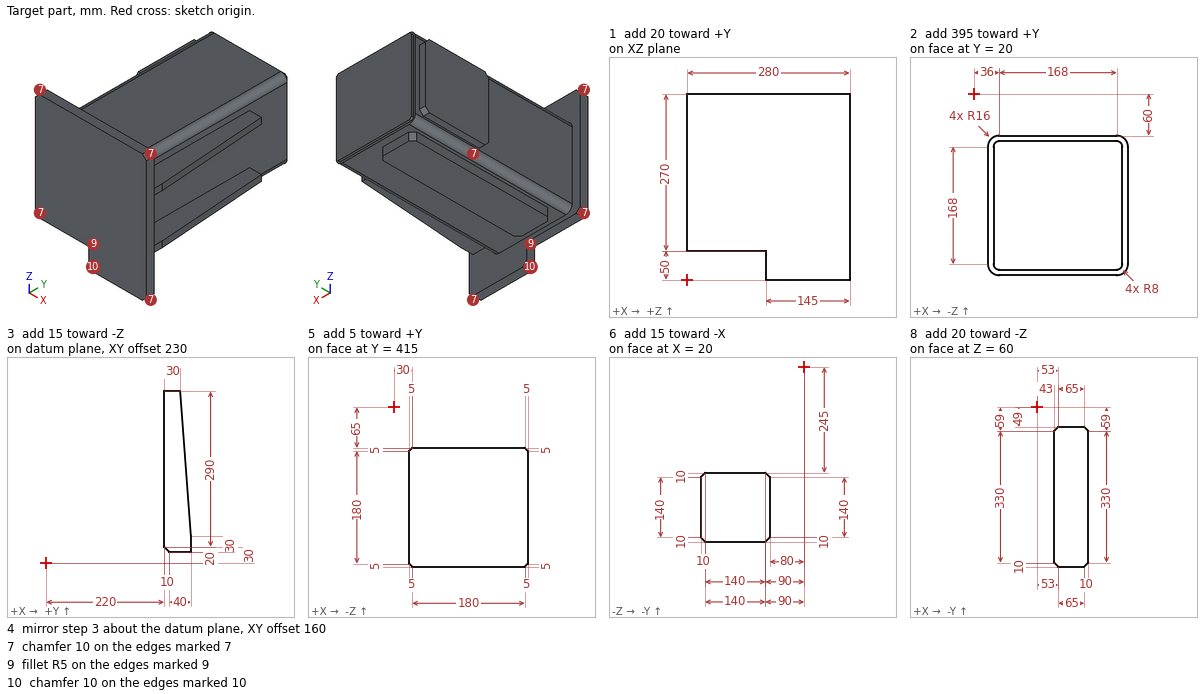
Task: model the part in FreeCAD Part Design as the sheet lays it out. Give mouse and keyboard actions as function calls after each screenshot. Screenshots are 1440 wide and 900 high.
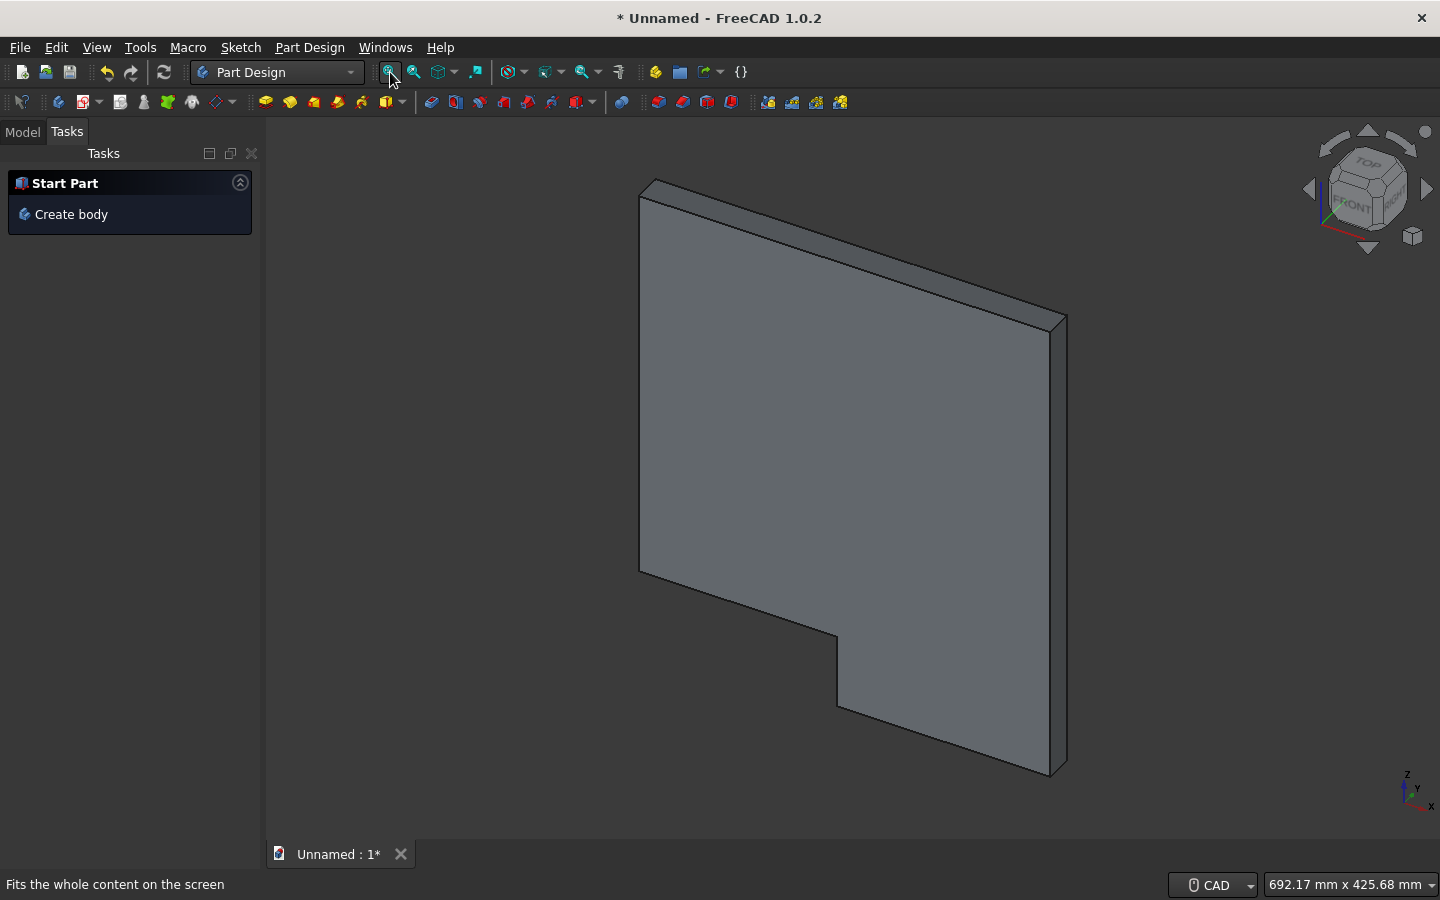
key(4)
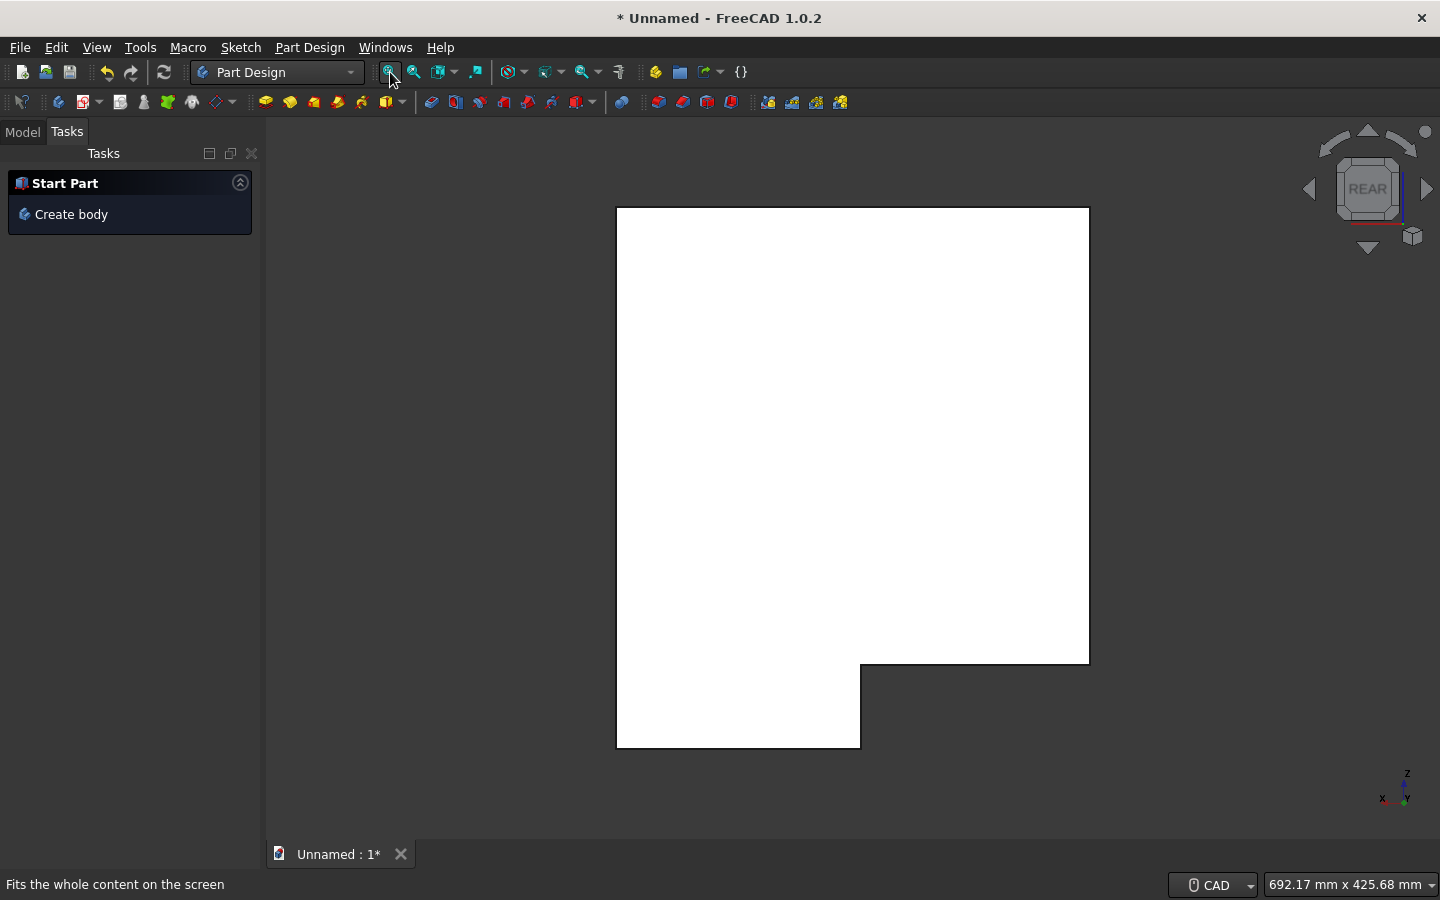
click(853, 399)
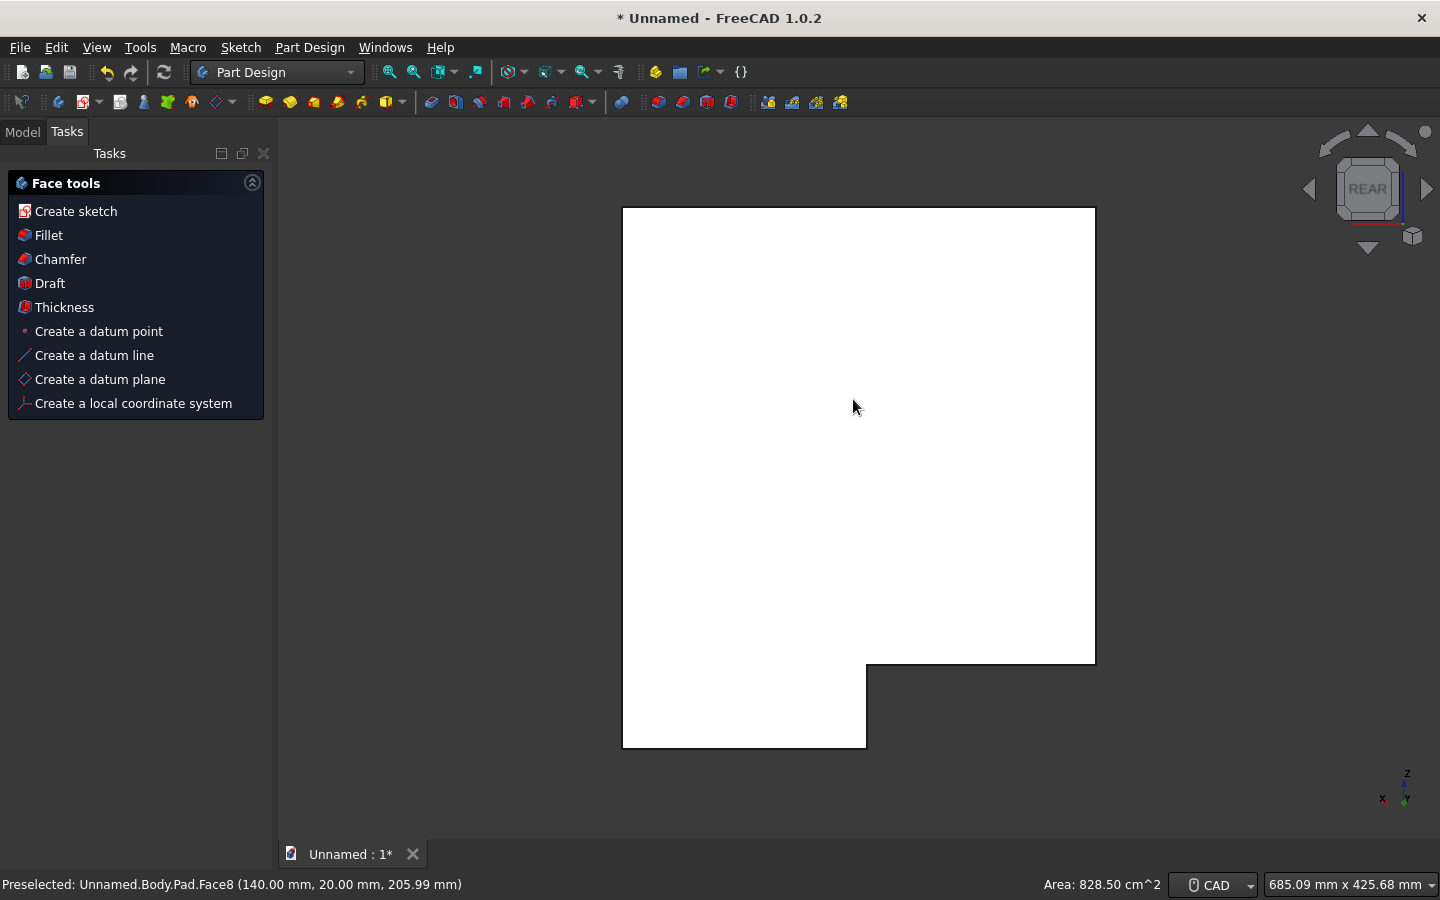
click(84, 102)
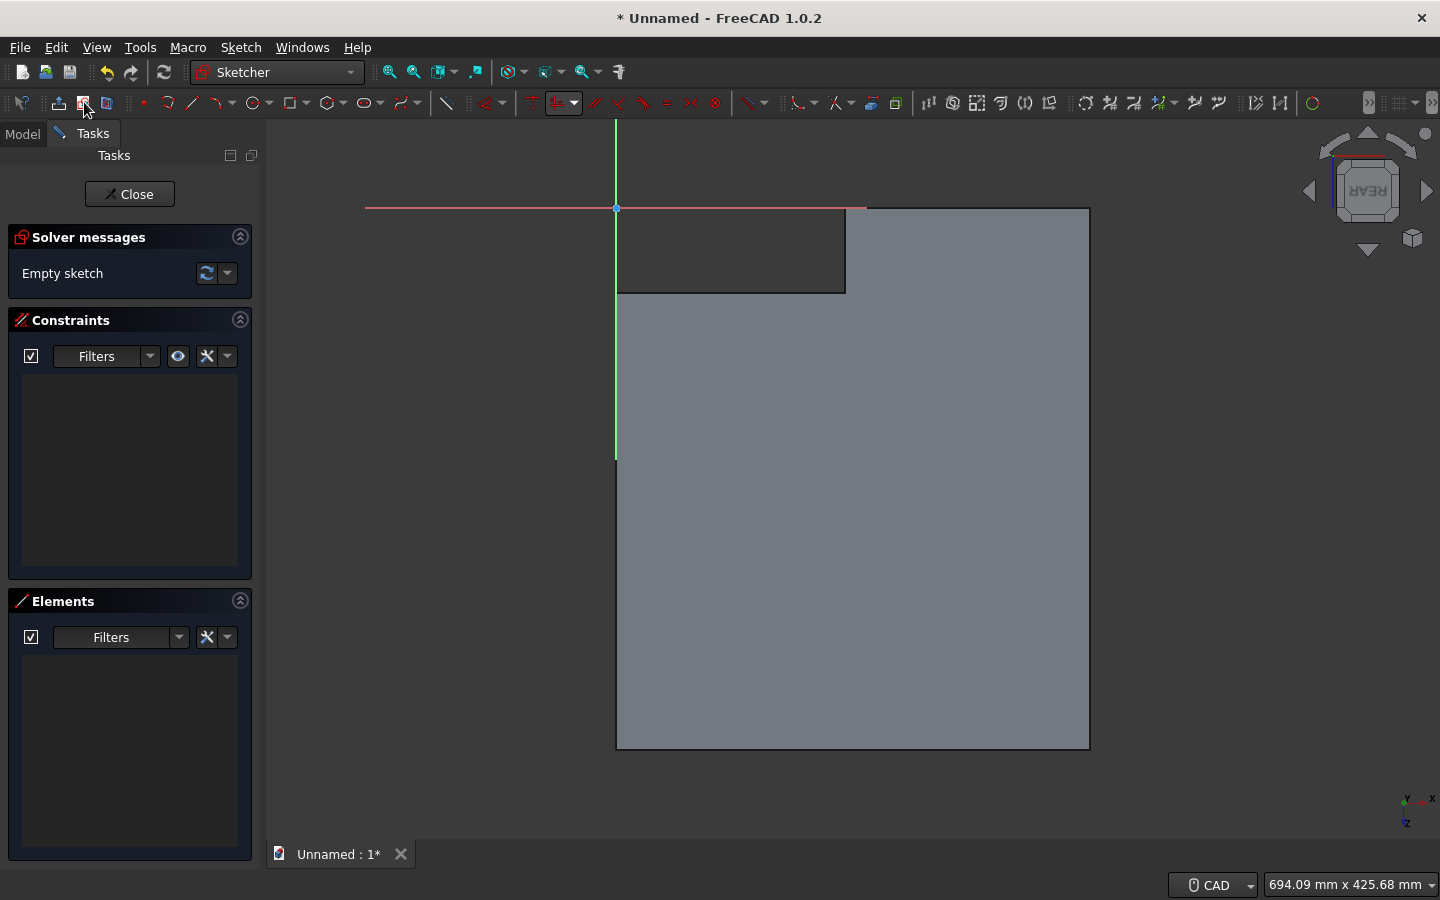
click(192, 104)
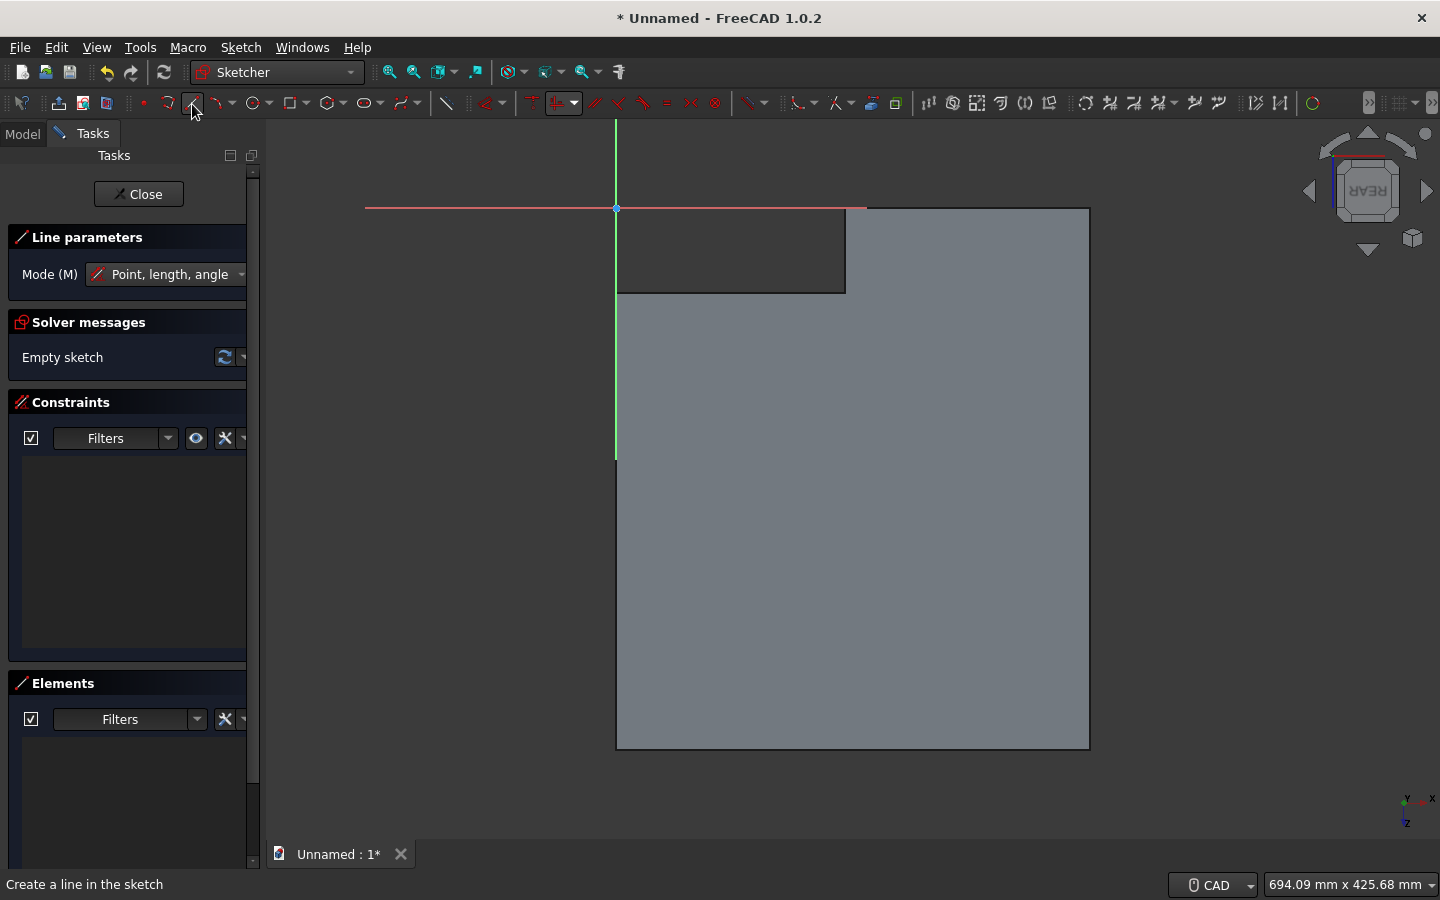
click(961, 310)
click(677, 310)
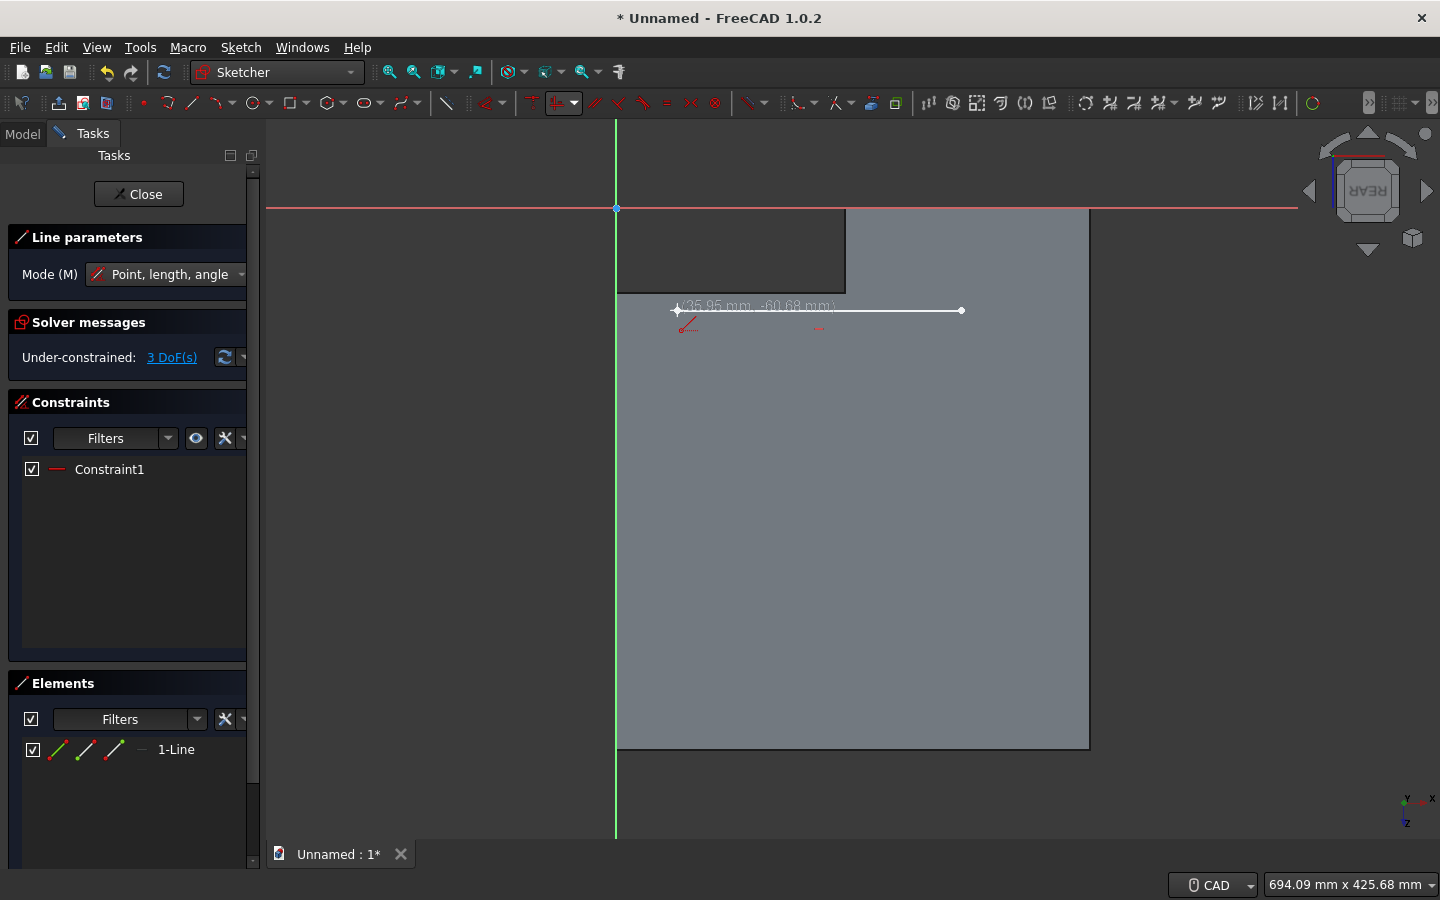
click(650, 337)
click(650, 621)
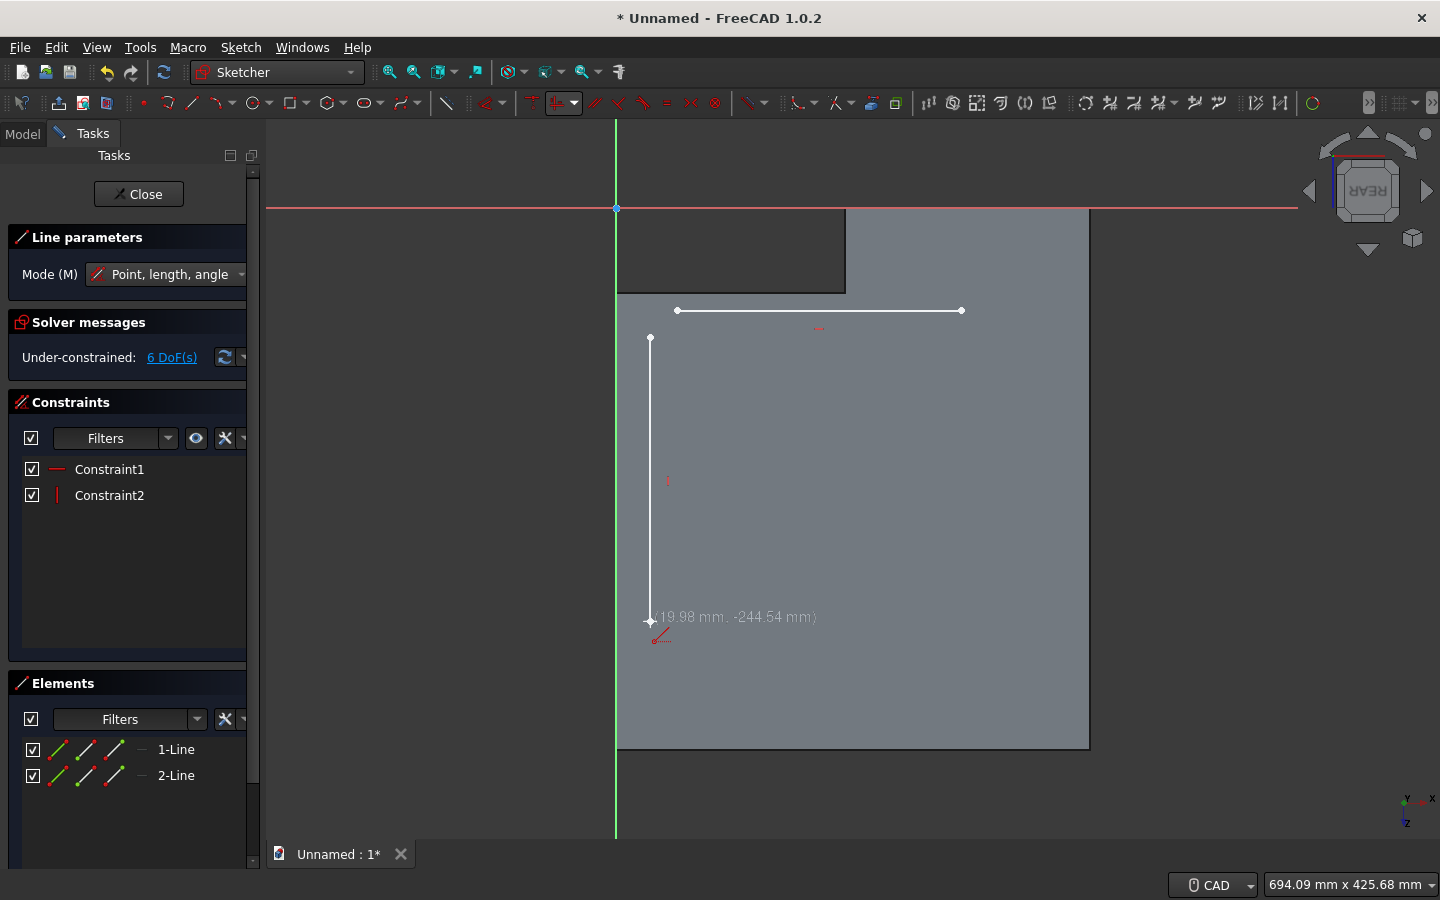
click(677, 648)
click(961, 648)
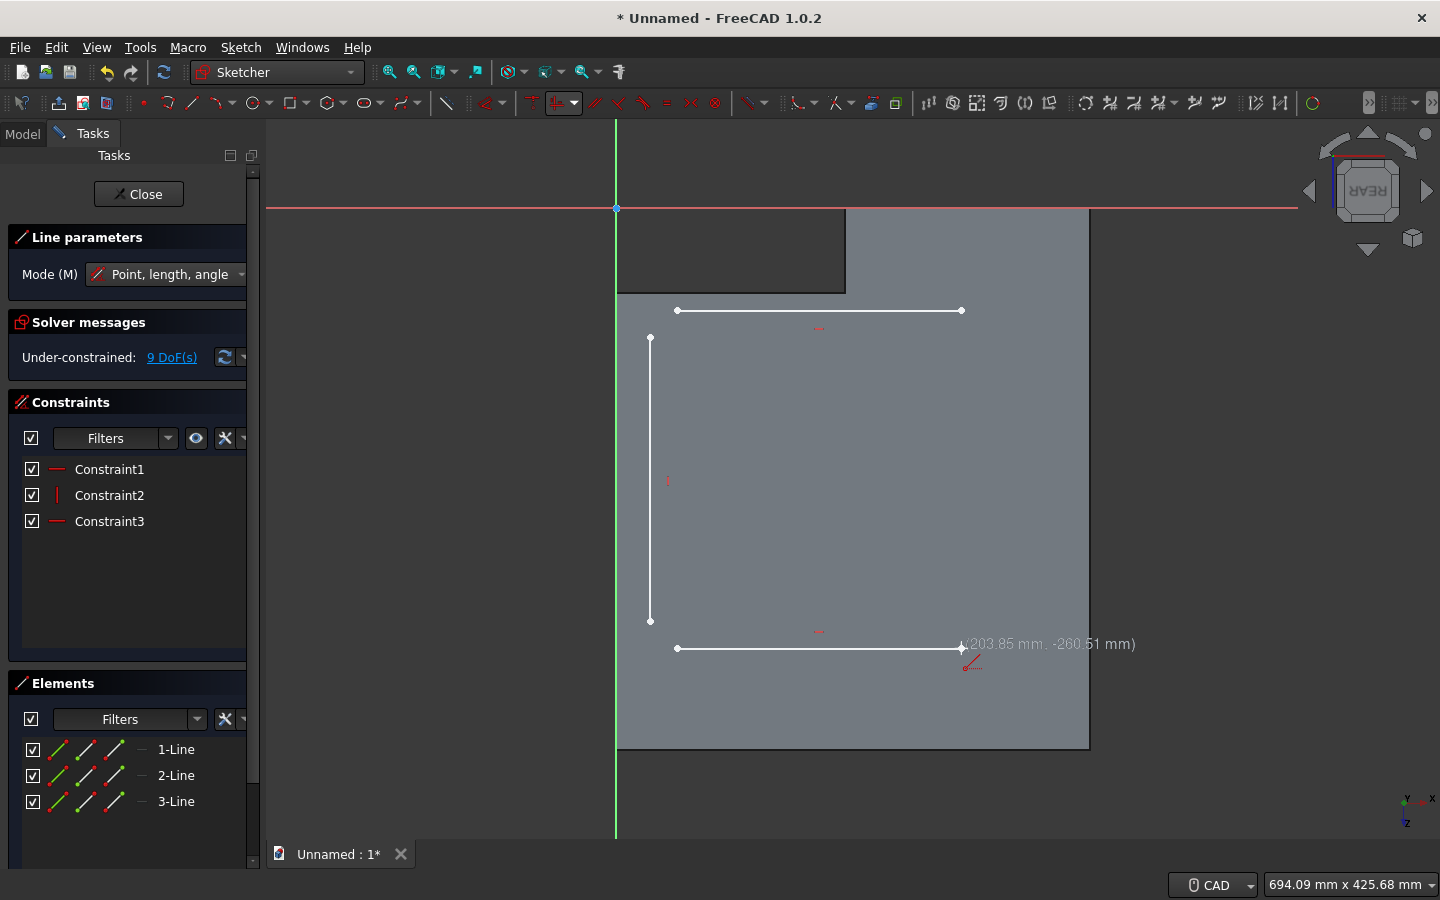
click(988, 621)
click(988, 337)